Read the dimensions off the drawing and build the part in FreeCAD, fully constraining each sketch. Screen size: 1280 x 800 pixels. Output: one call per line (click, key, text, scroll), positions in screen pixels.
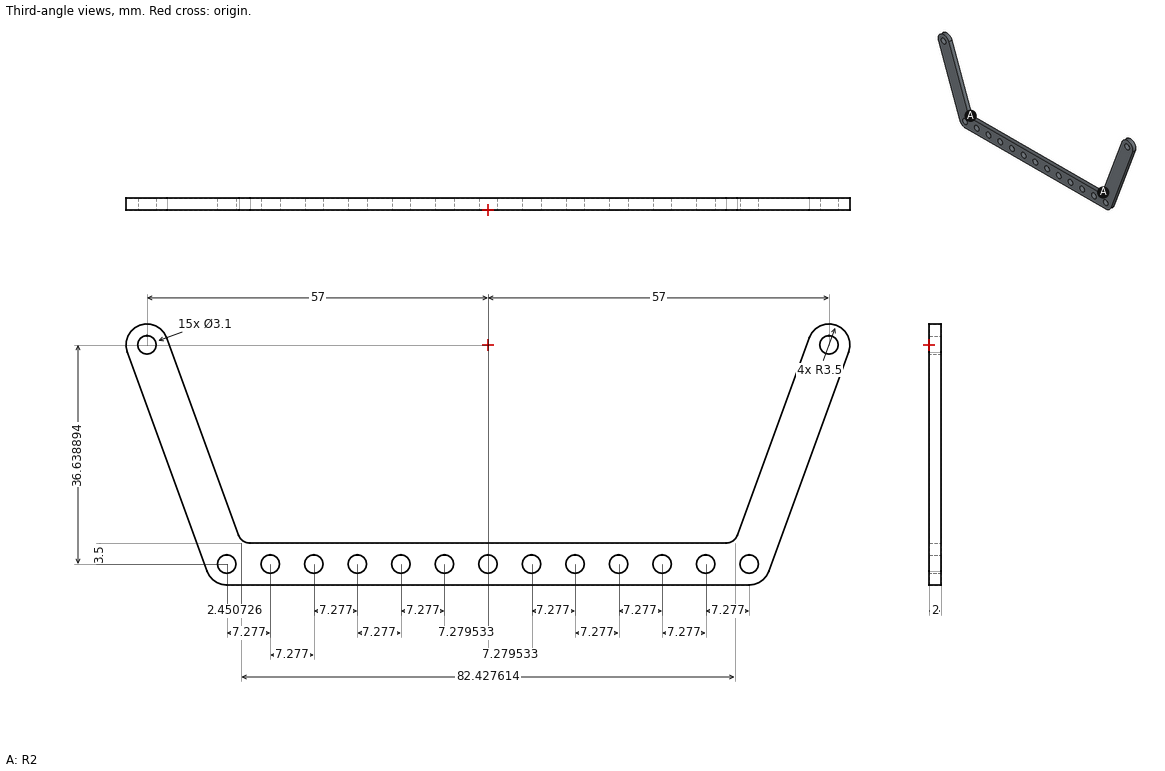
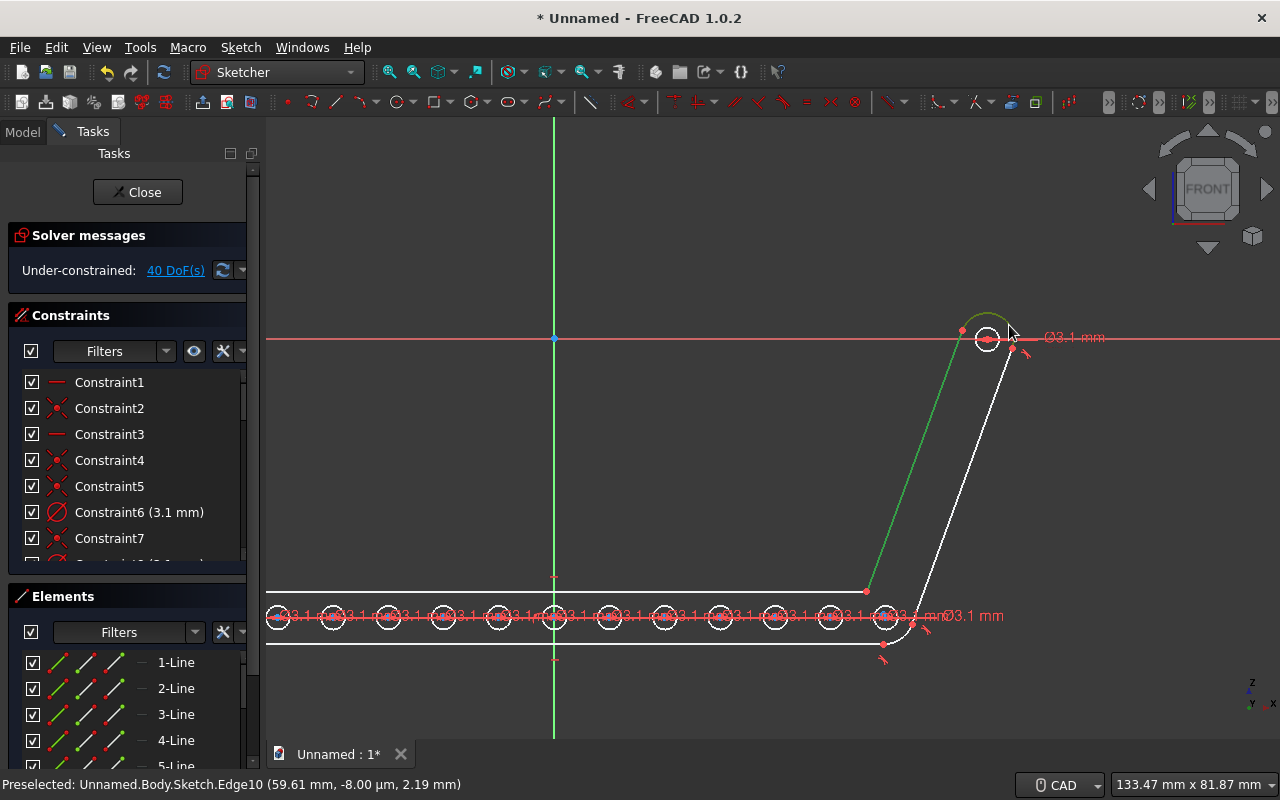
key(t)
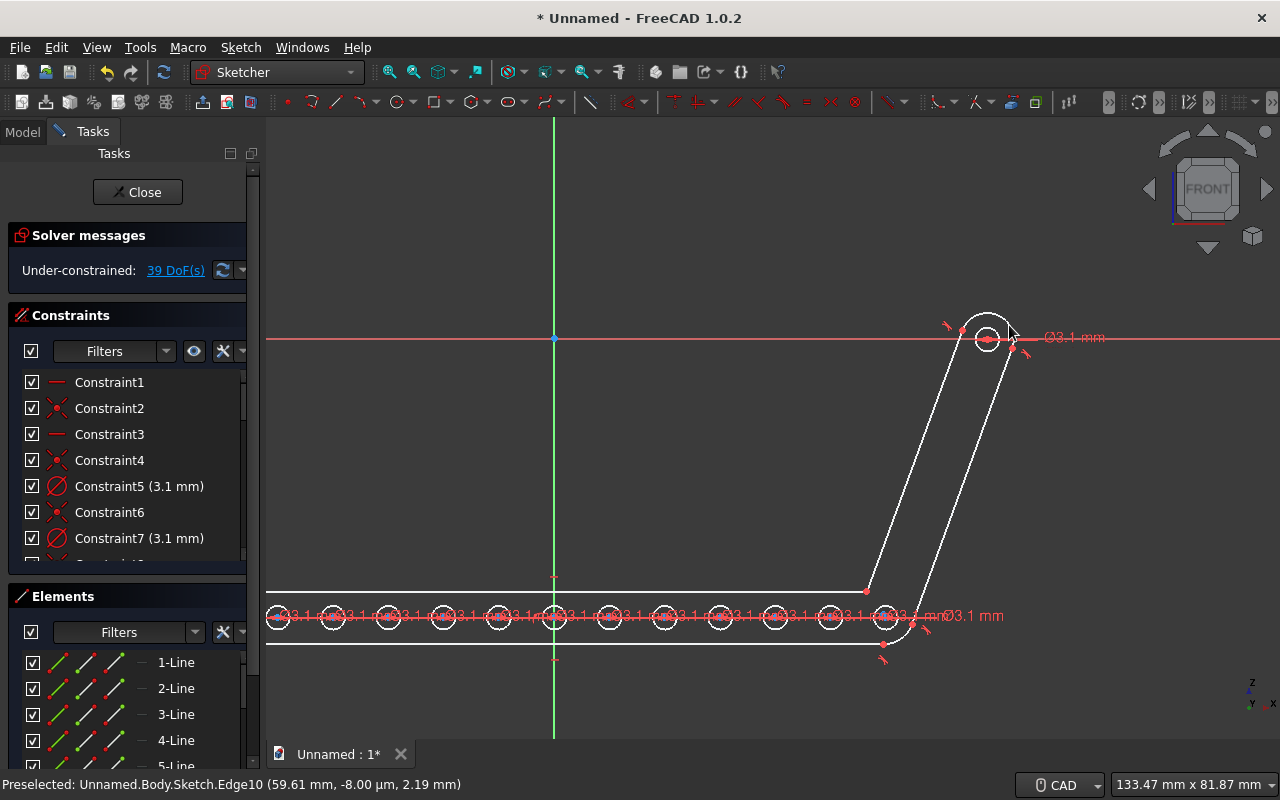
click(894, 609)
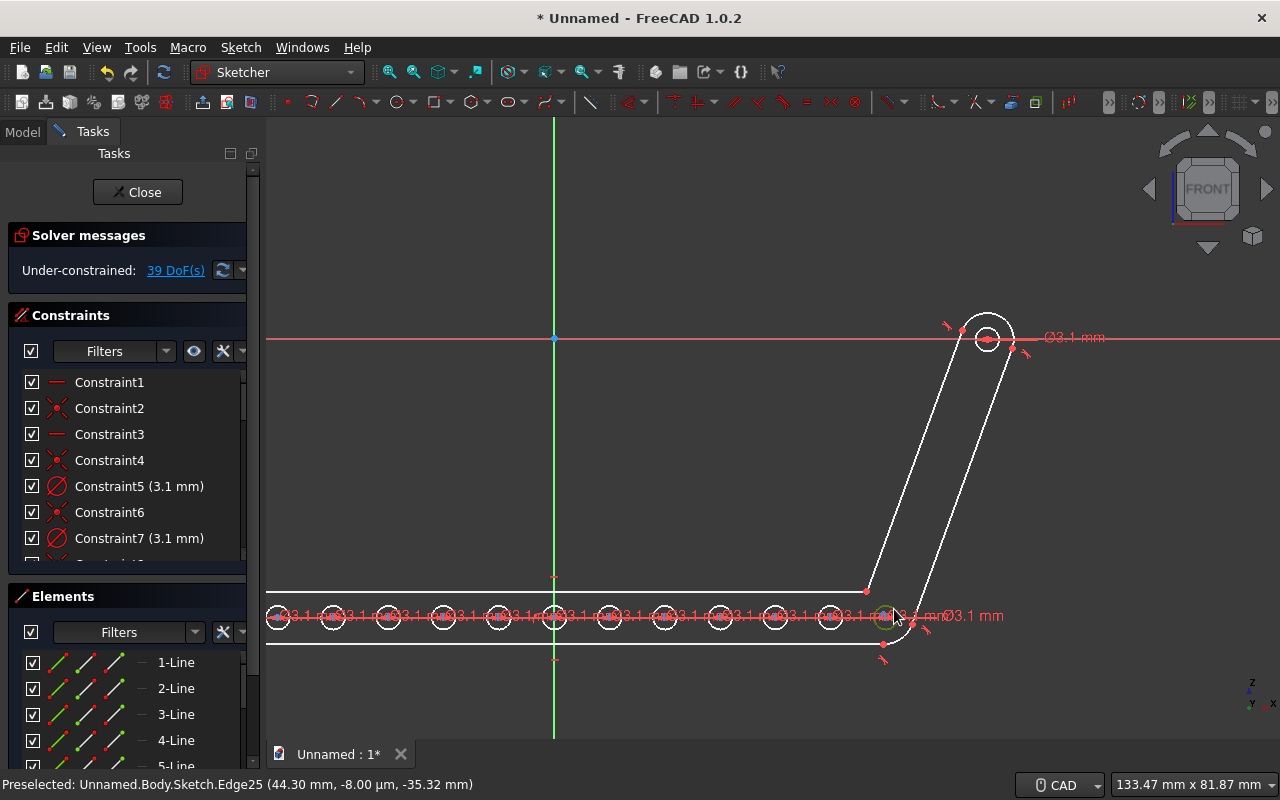
scroll(894, 642, up, 2)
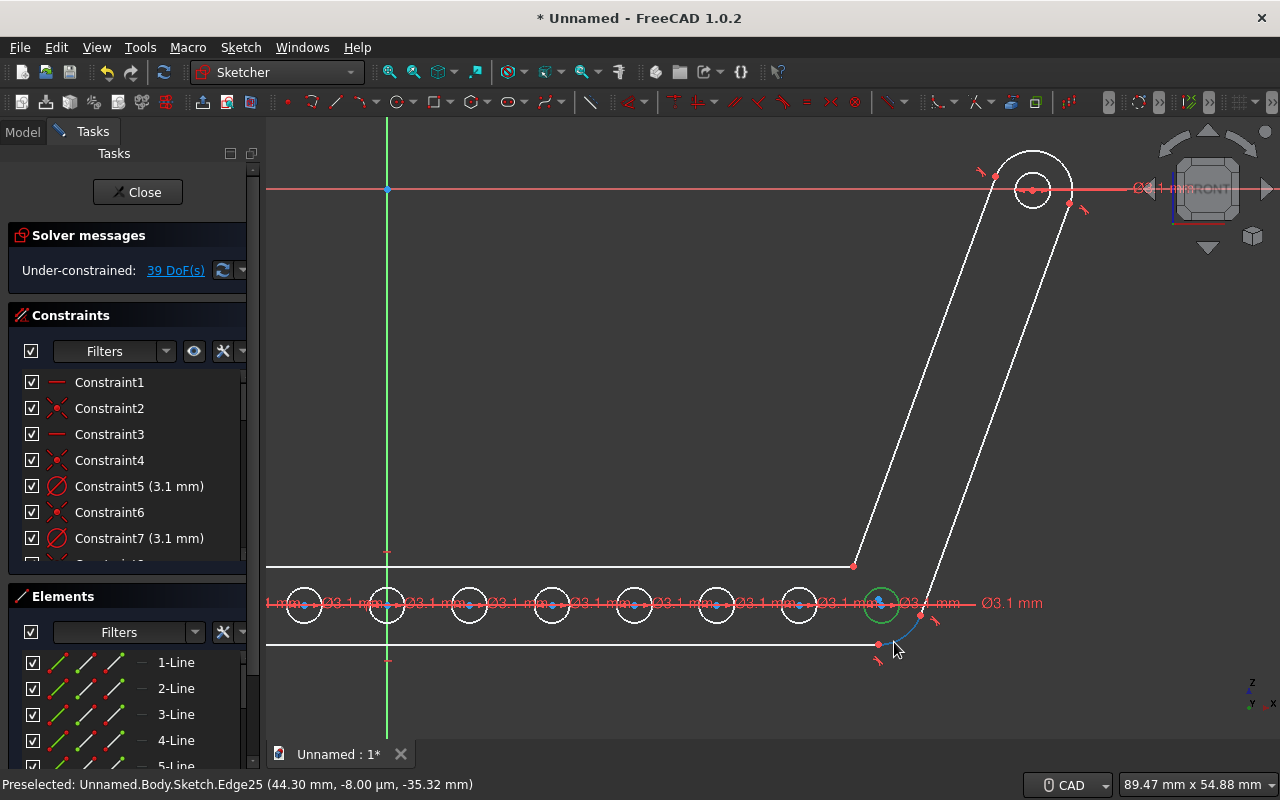
click(894, 642)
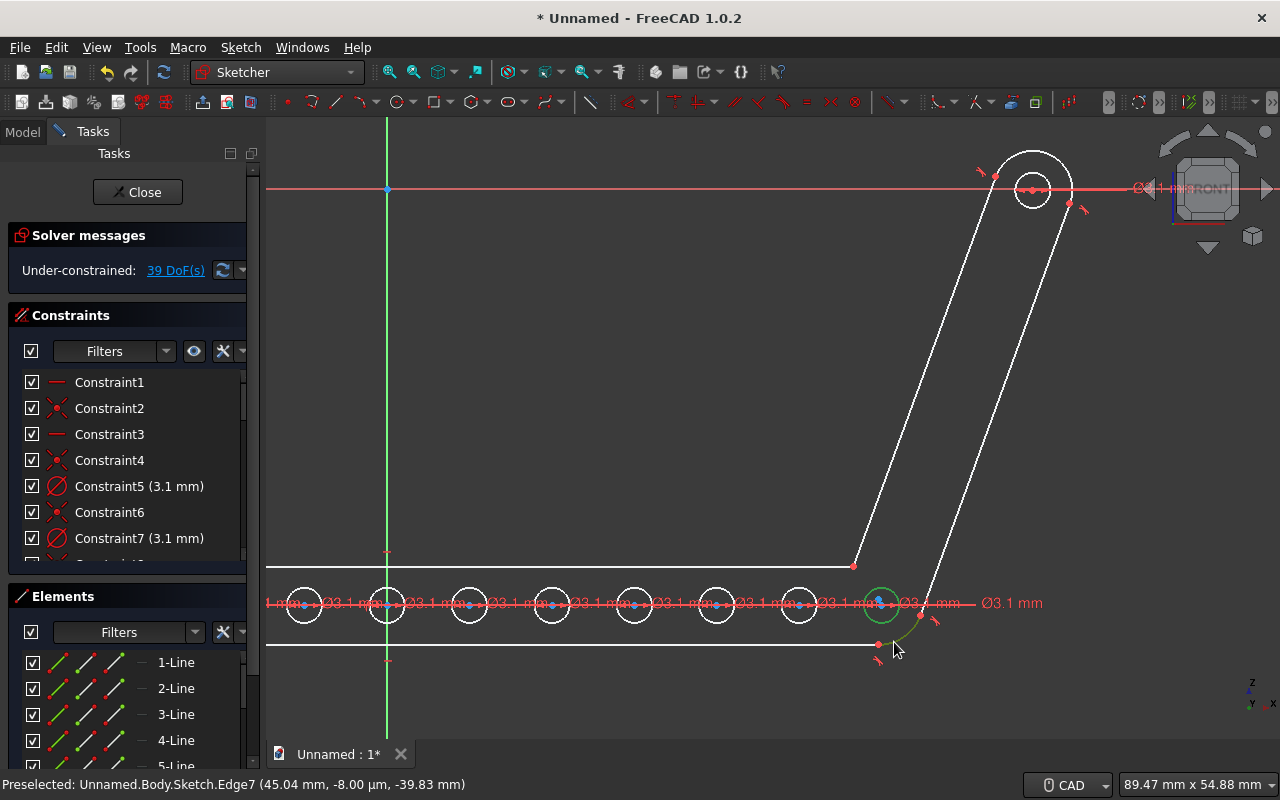
key(c)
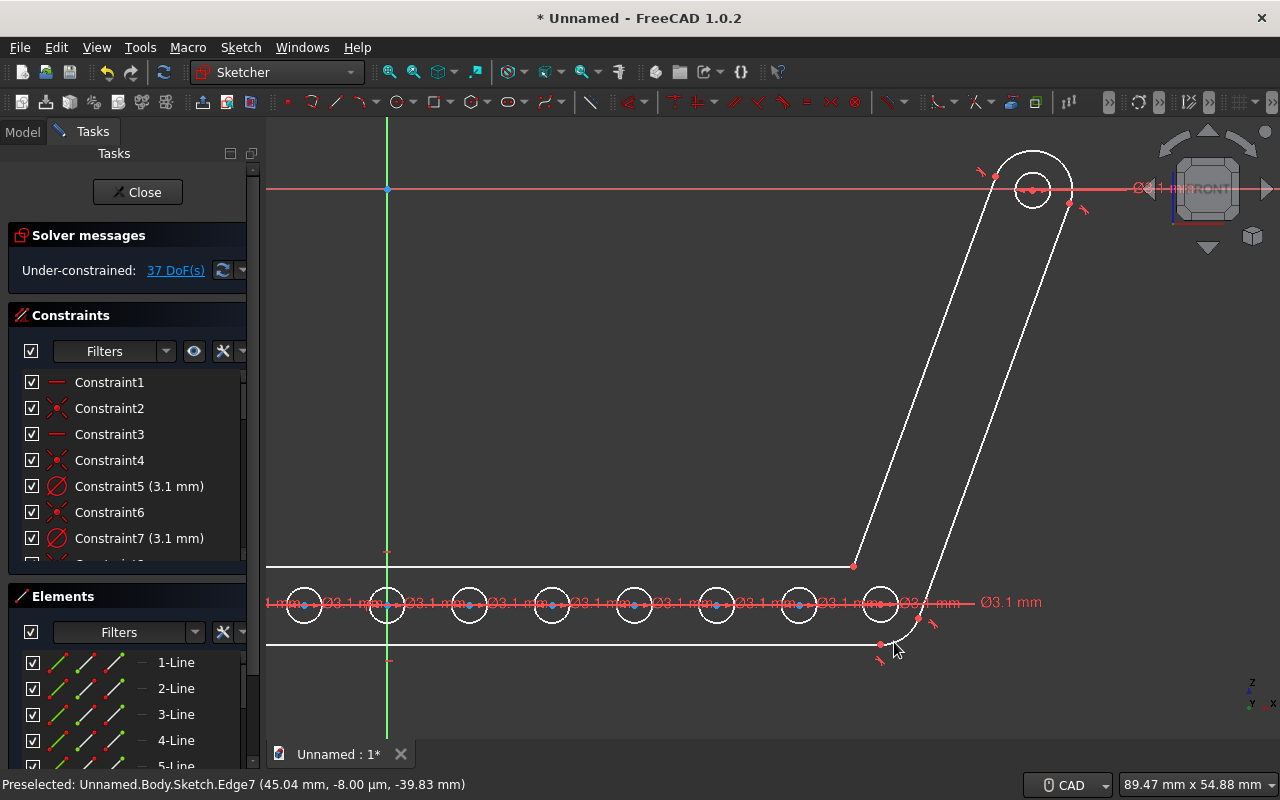
scroll(964, 452, down, 4)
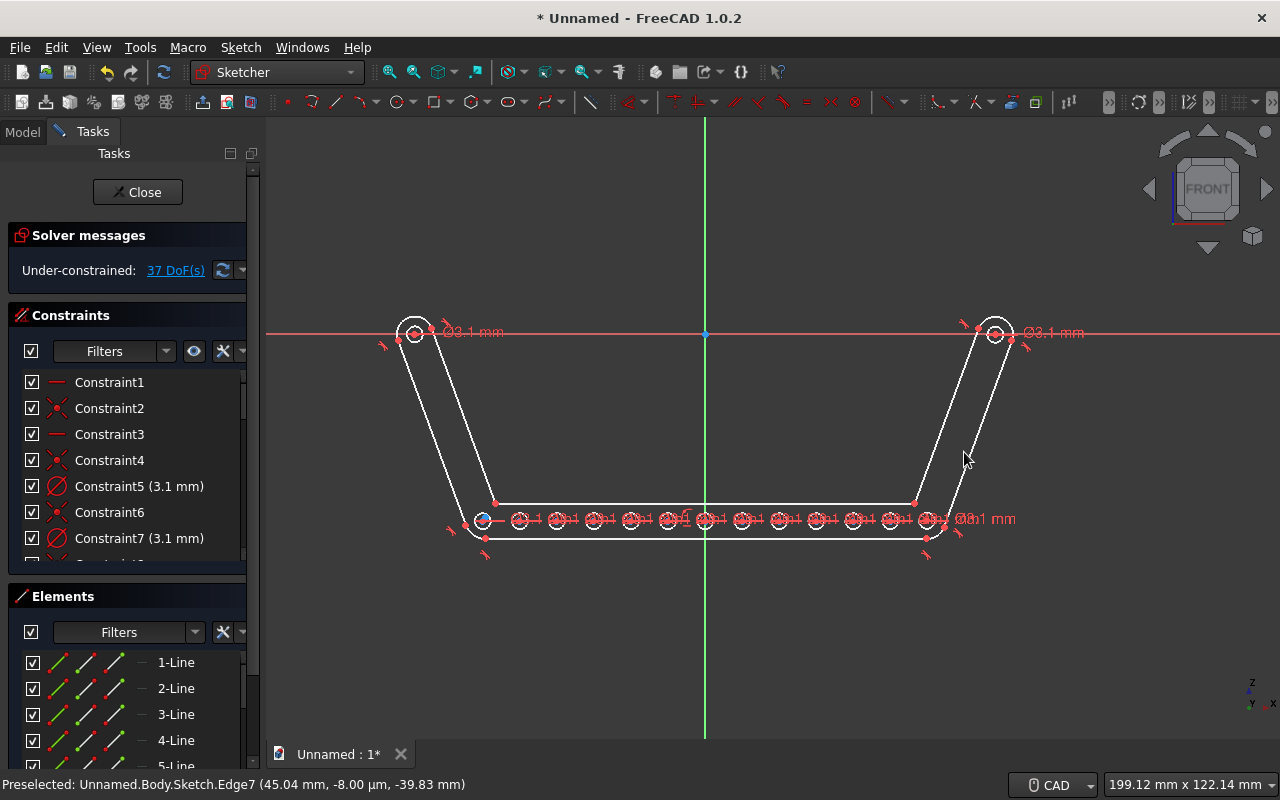
scroll(488, 516, up, 3)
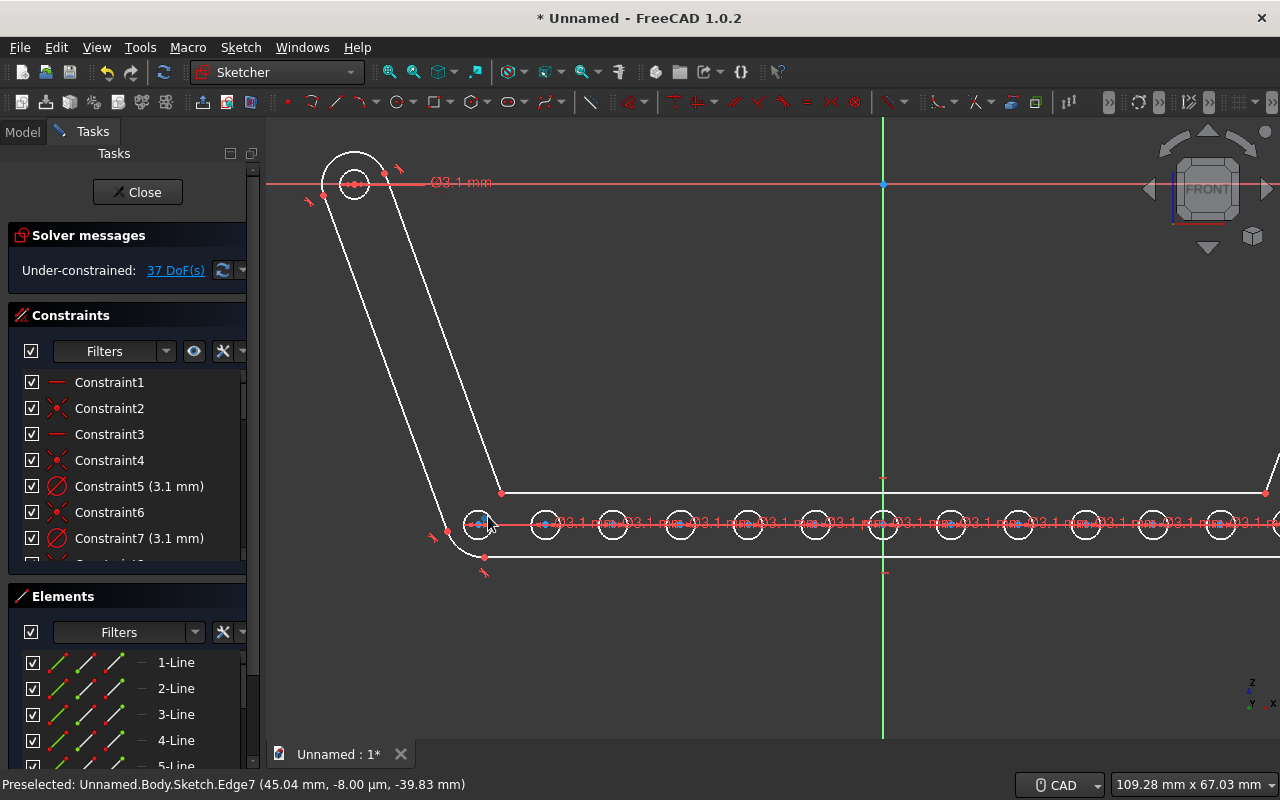
click(468, 515)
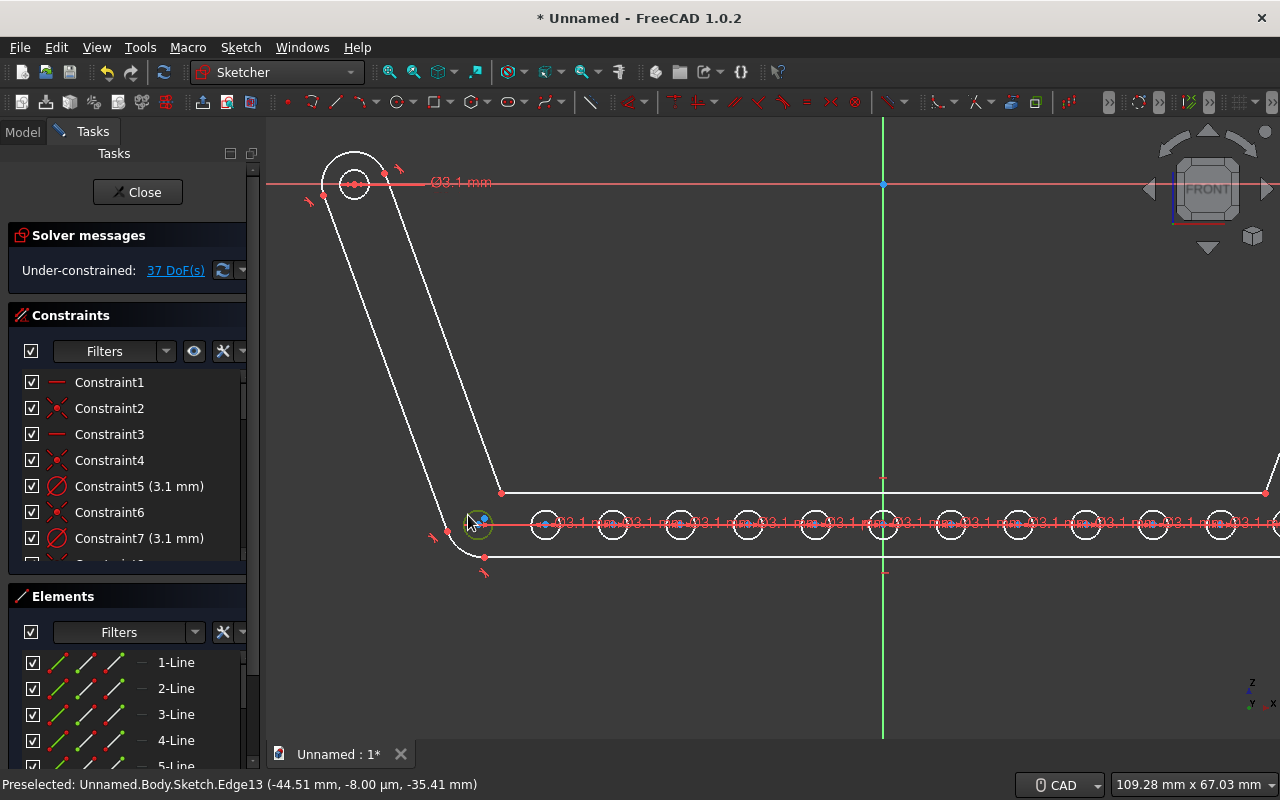
click(455, 544)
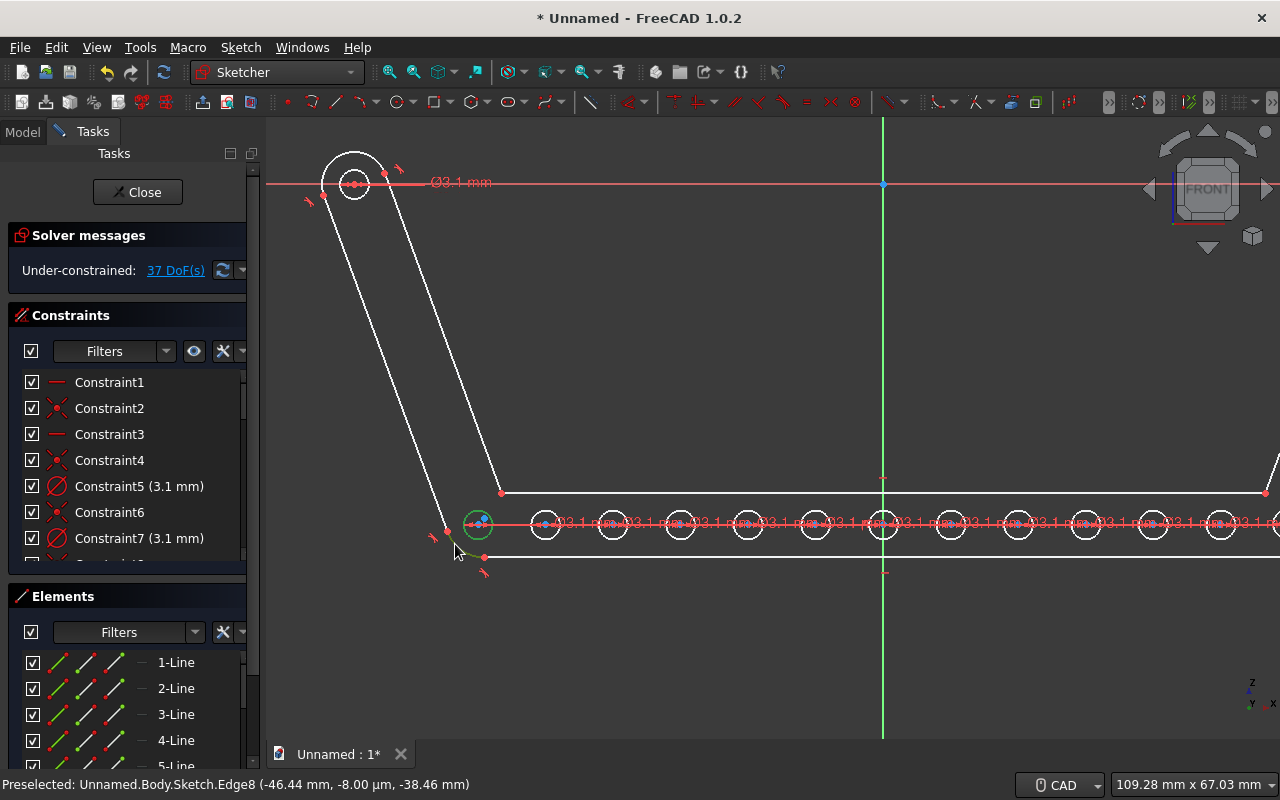
click(674, 102)